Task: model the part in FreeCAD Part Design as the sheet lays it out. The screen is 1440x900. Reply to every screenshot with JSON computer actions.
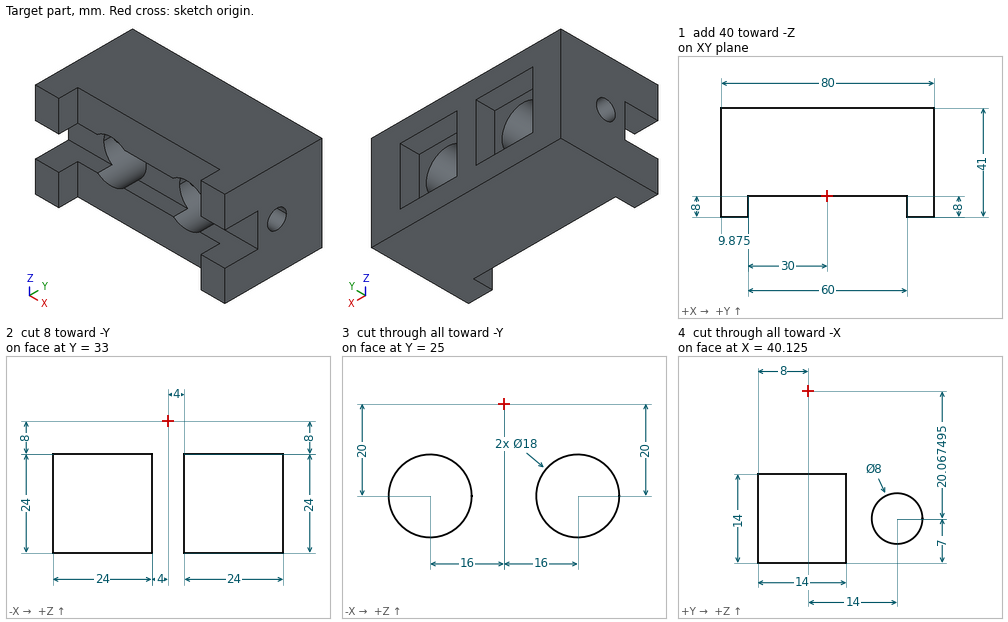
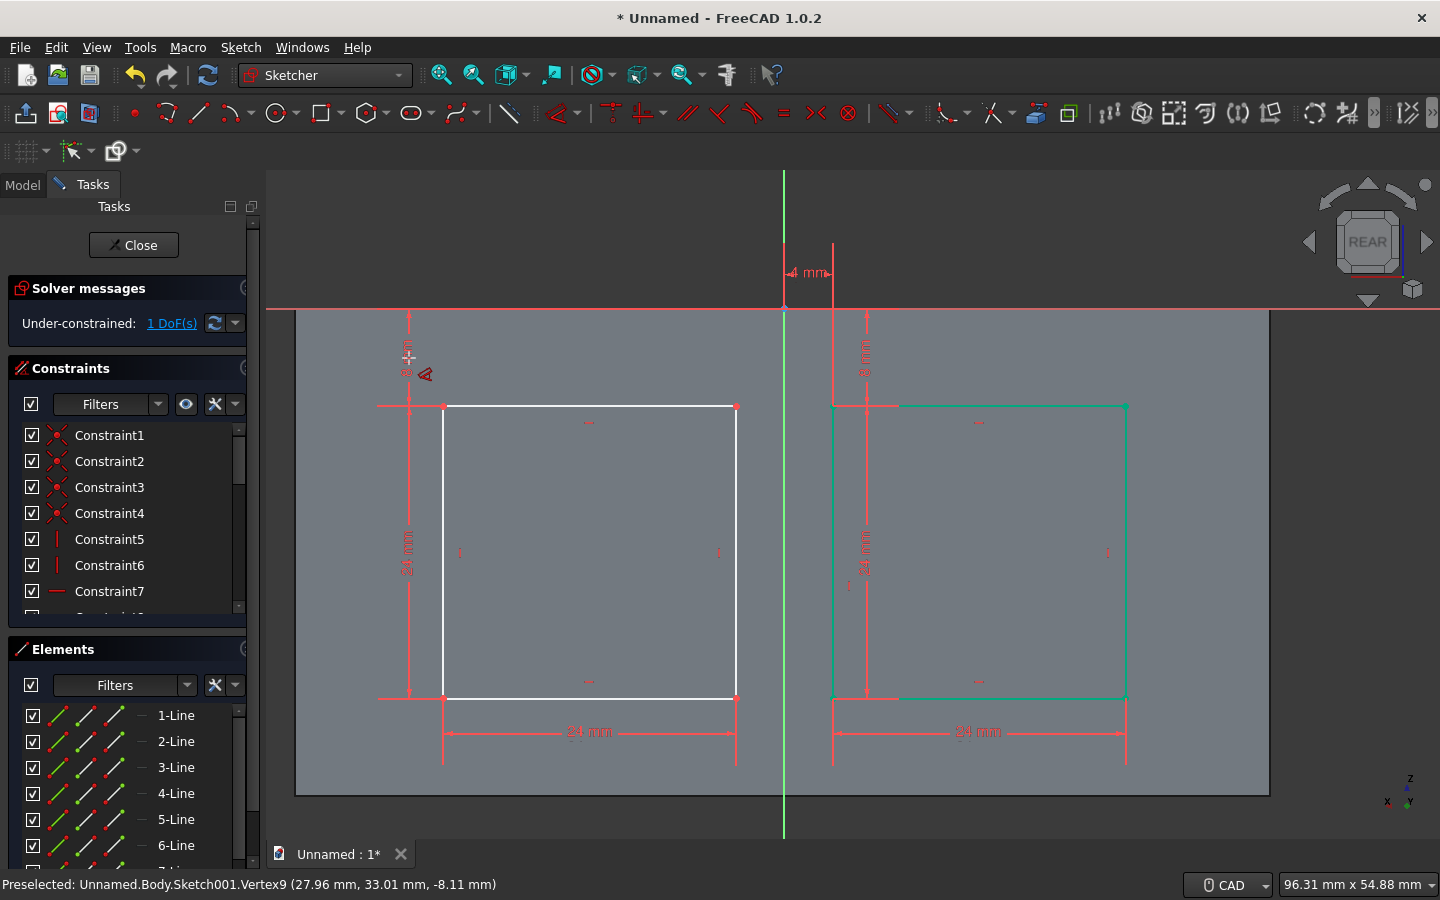
{"action": "left_click", "coordinate": [736, 699]}
{"action": "left_click", "coordinate": [760, 733]}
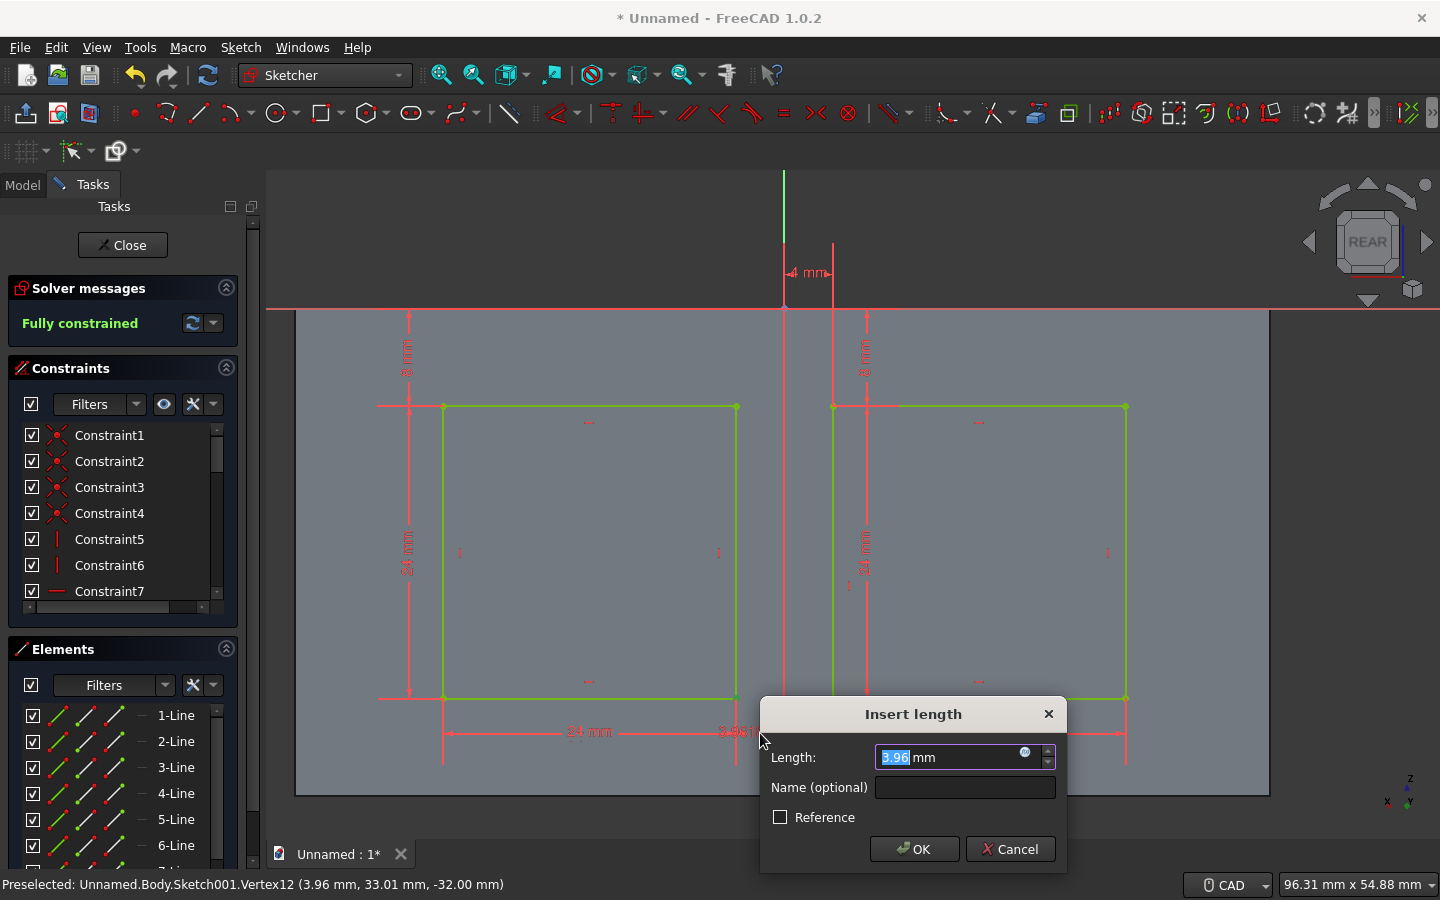
{"action": "type", "text": "4"}
{"action": "key", "text": "Return"}
{"action": "key", "text": "Escape"}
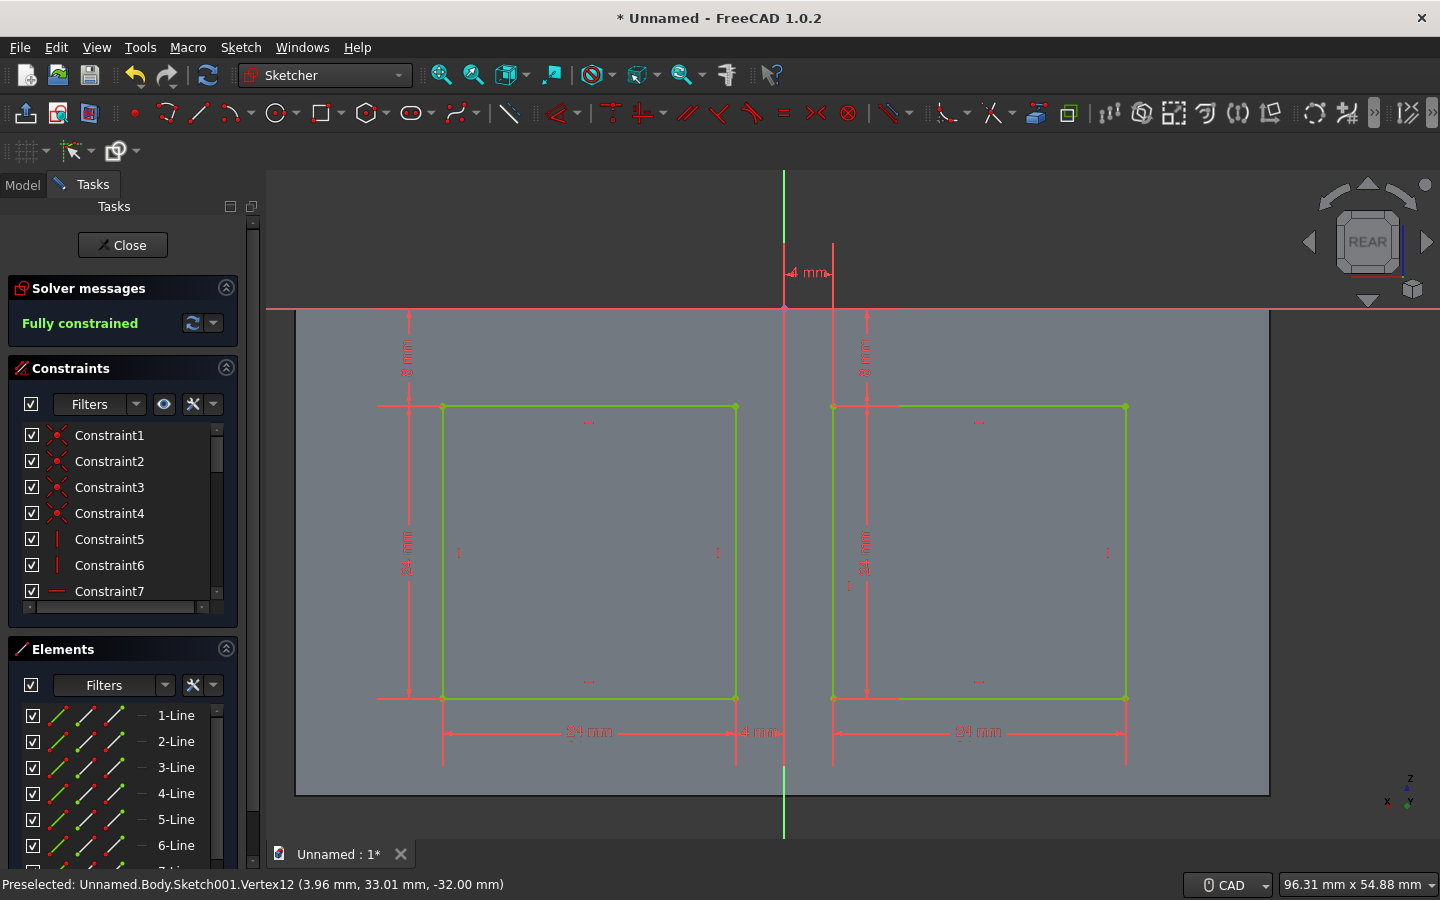
{"action": "left_click", "coordinate": [123, 245]}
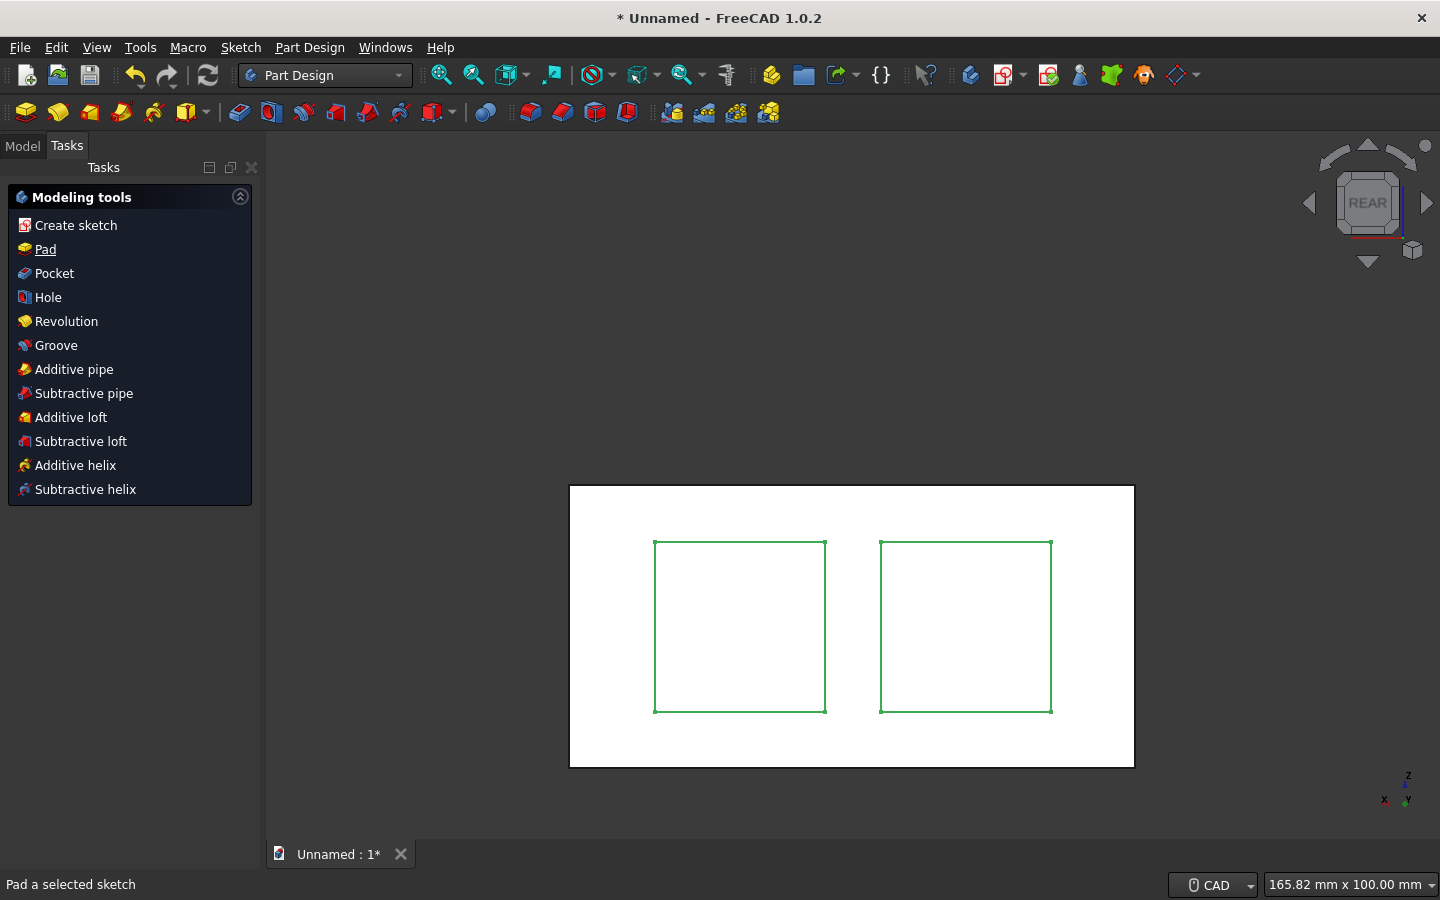
{"action": "left_click", "coordinate": [240, 112]}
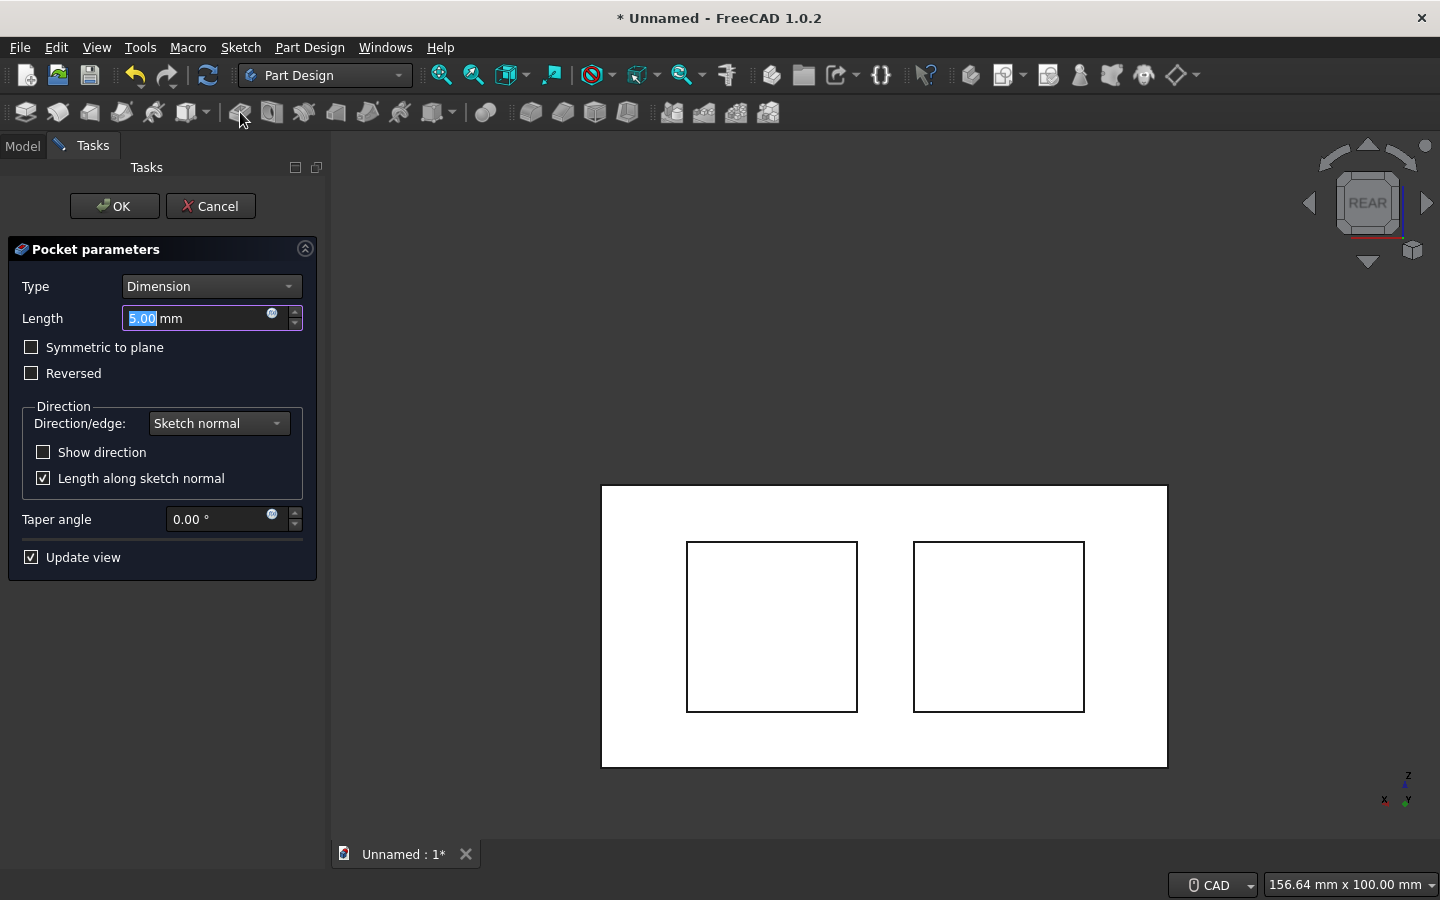
{"action": "type", "text": "8"}
{"action": "key", "text": "Tab"}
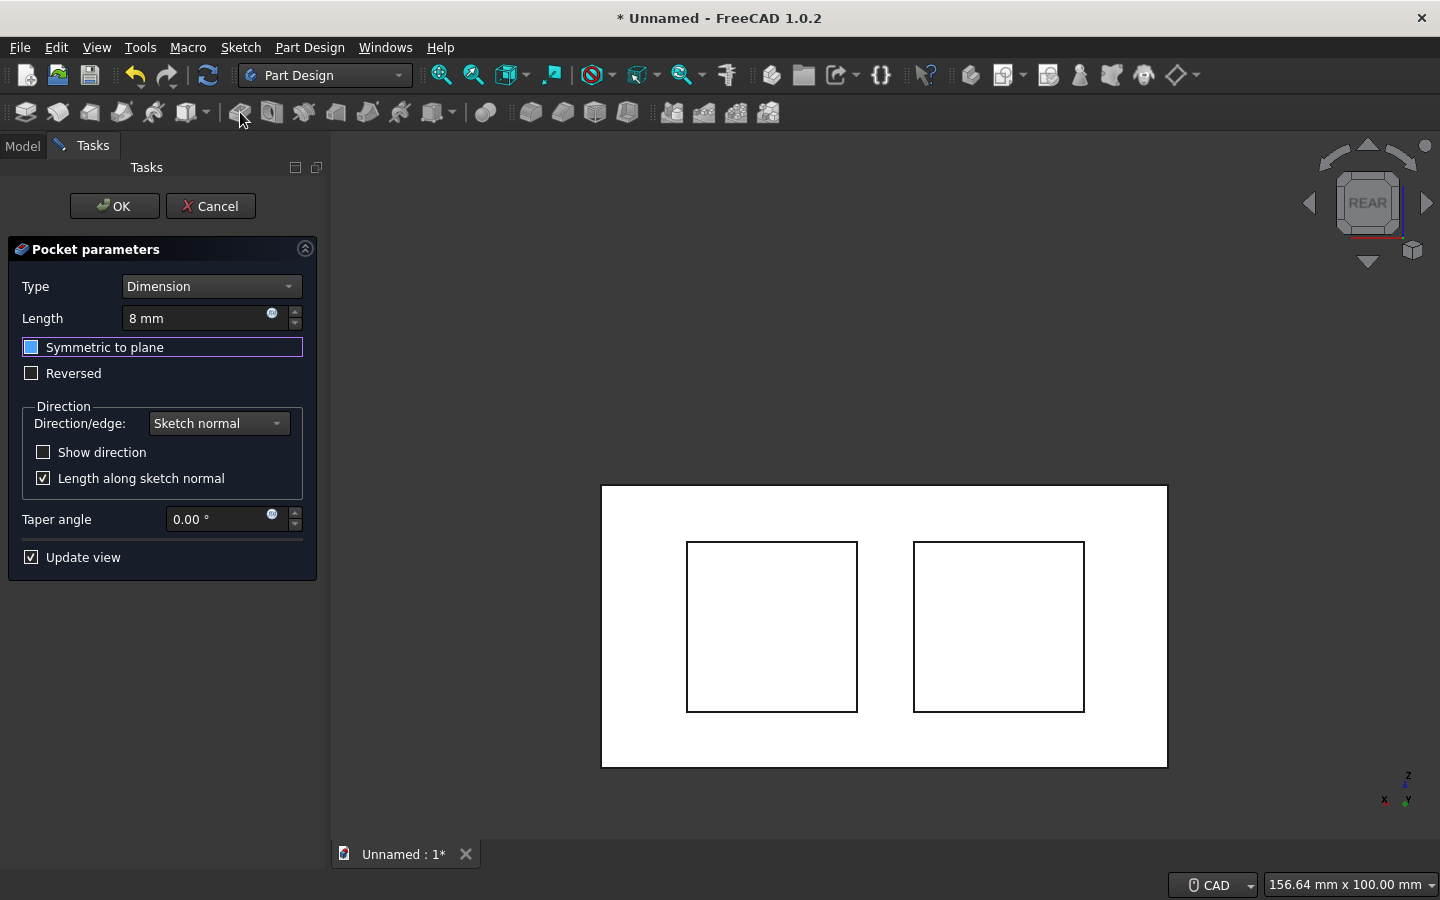
{"action": "left_click", "coordinate": [115, 206]}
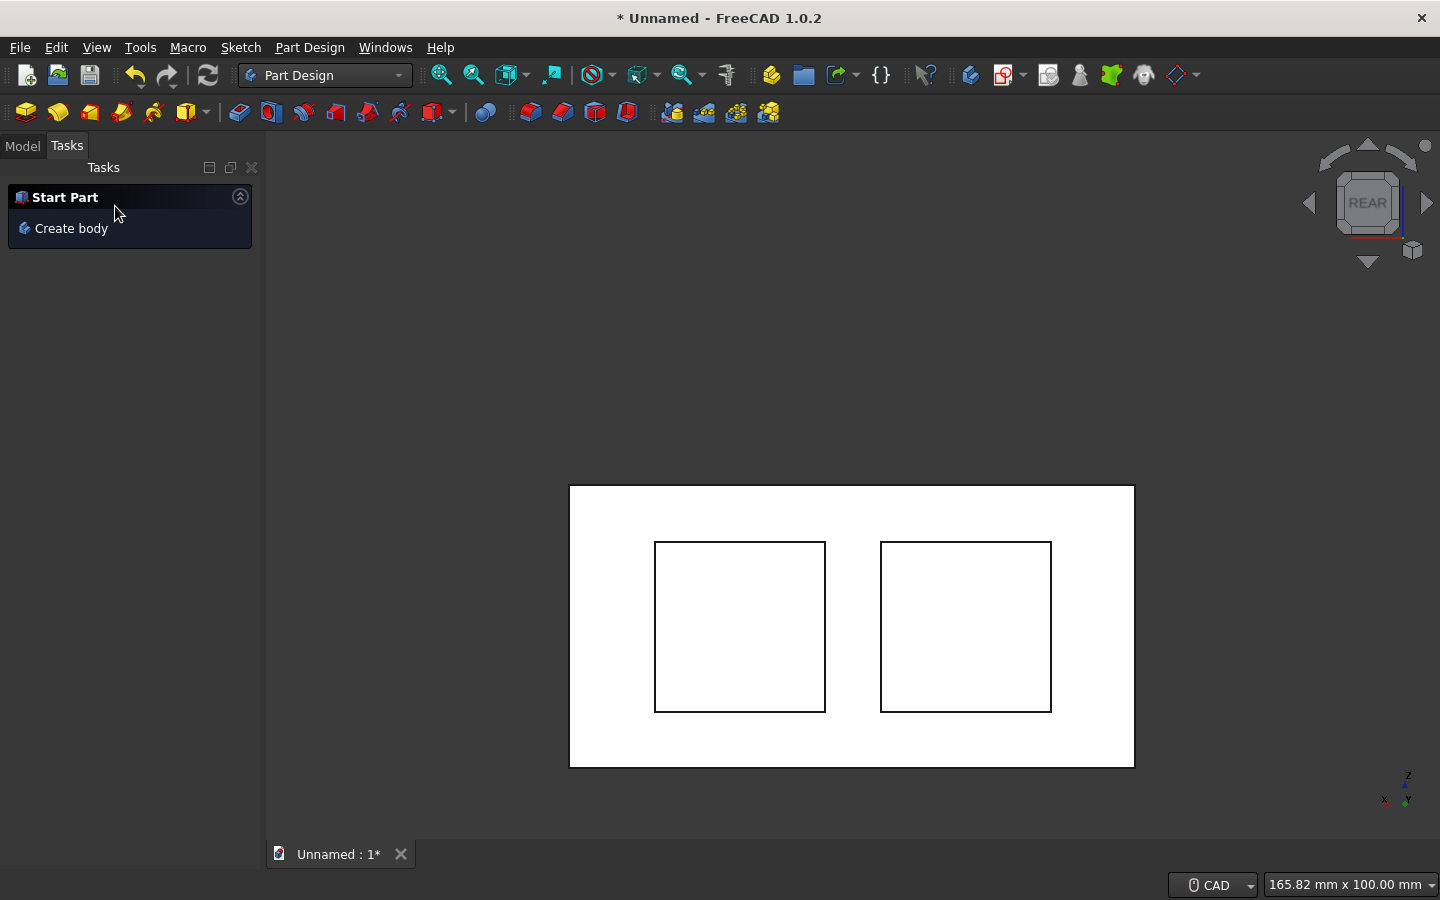
{"action": "left_click", "coordinate": [966, 626]}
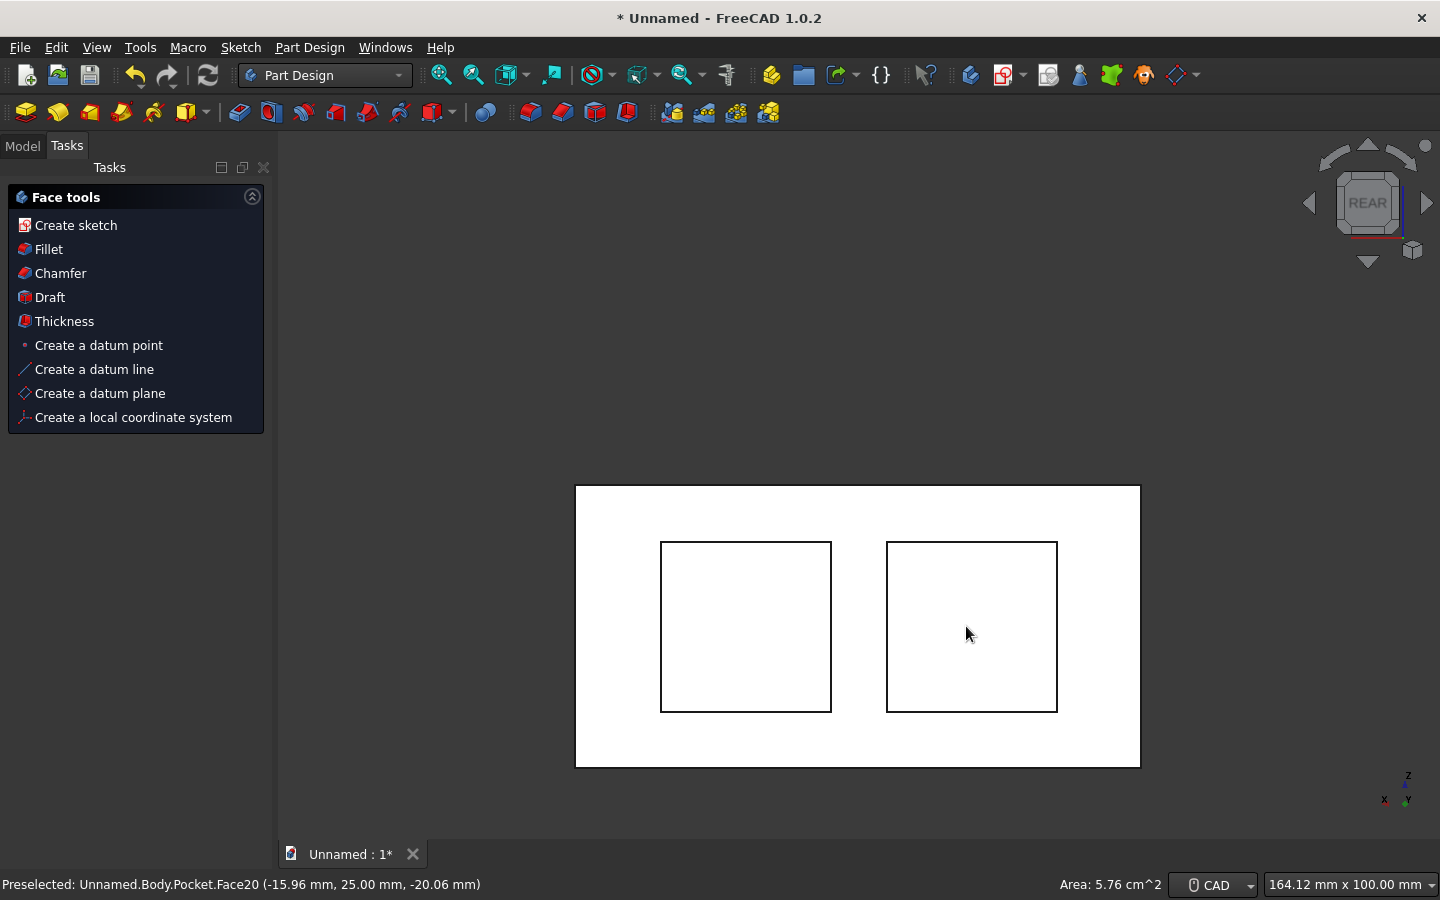
{"action": "left_click", "coordinate": [1004, 76]}